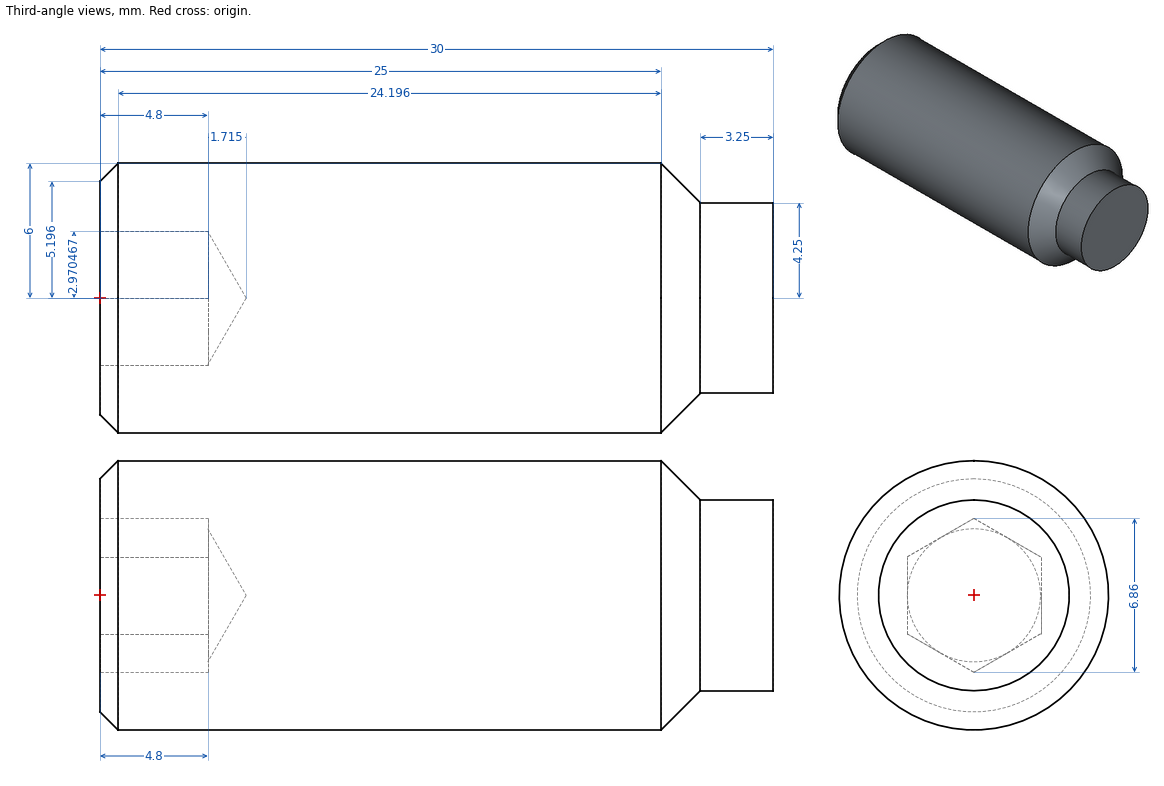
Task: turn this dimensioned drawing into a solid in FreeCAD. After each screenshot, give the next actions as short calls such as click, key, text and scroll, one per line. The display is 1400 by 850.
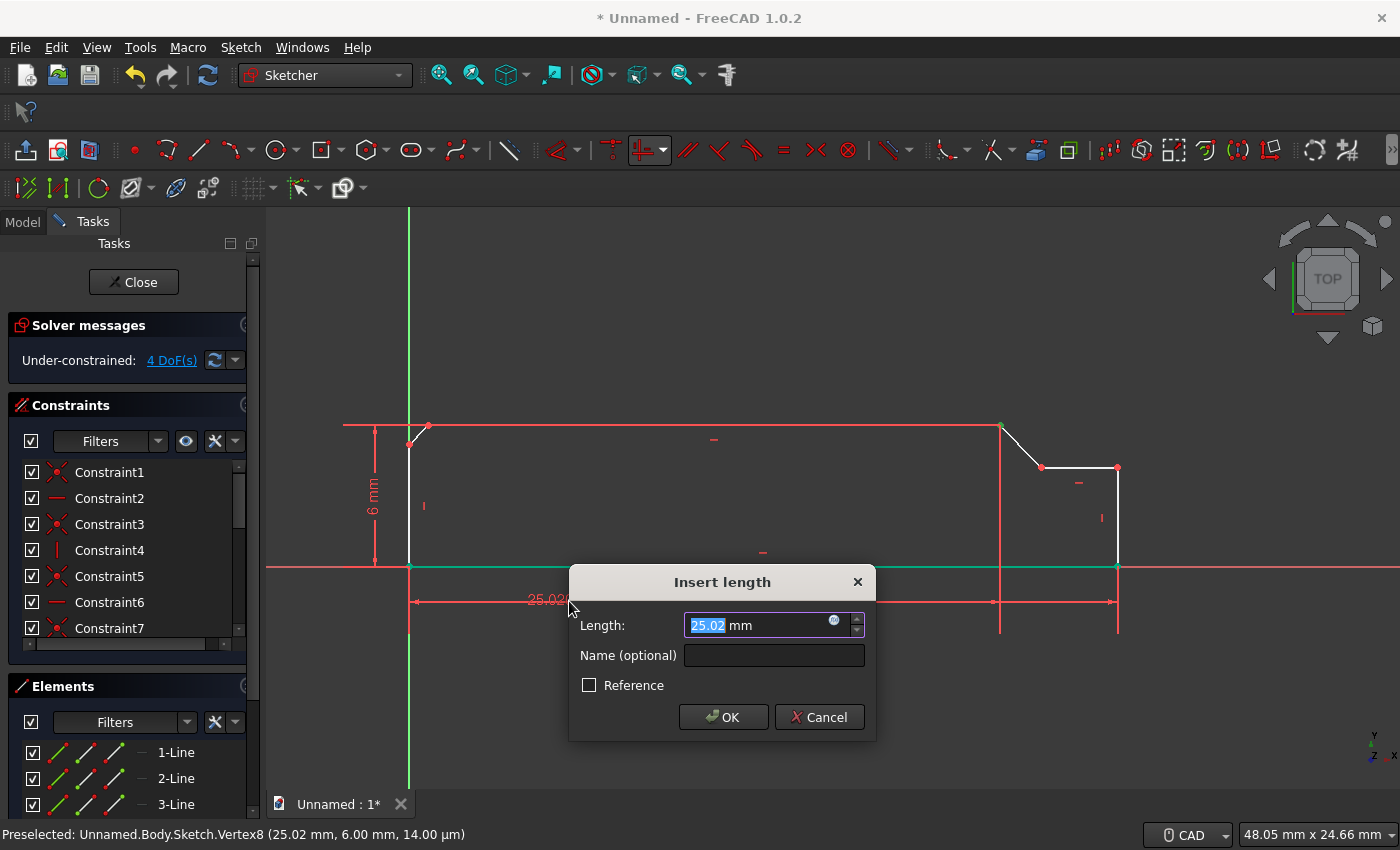
text(25)
key(Return)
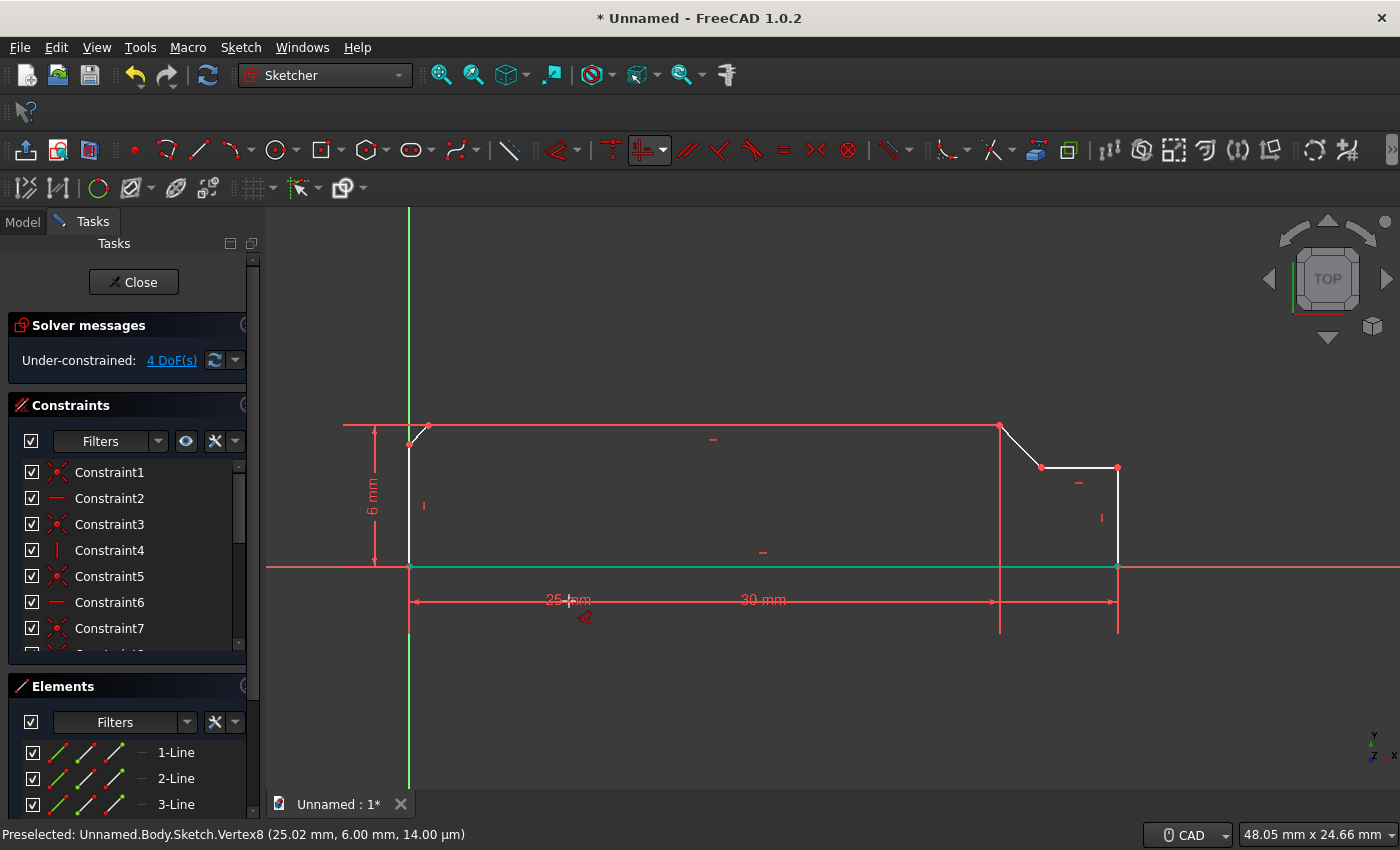
click(1118, 537)
click(1152, 517)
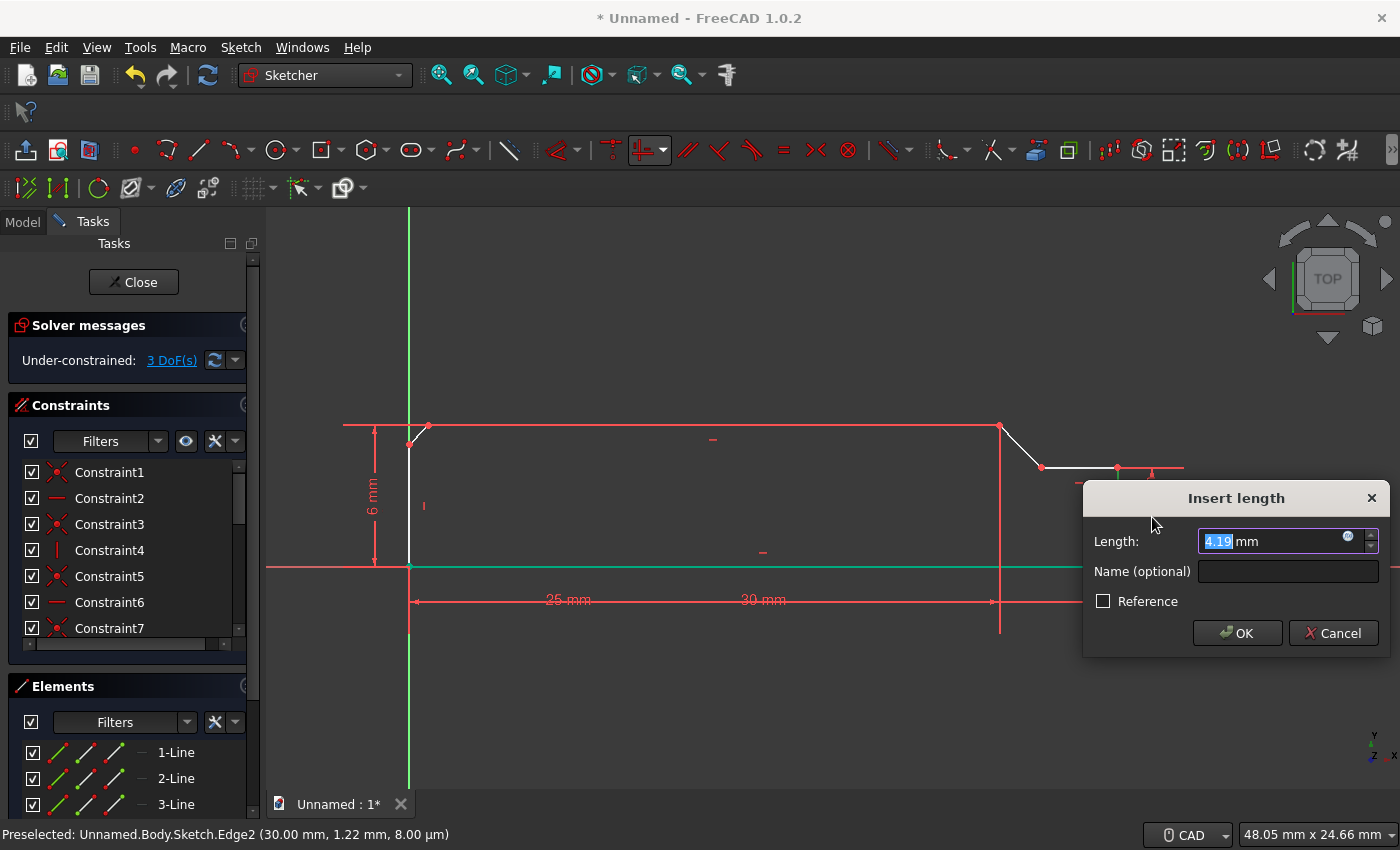
text(4.25)
key(Return)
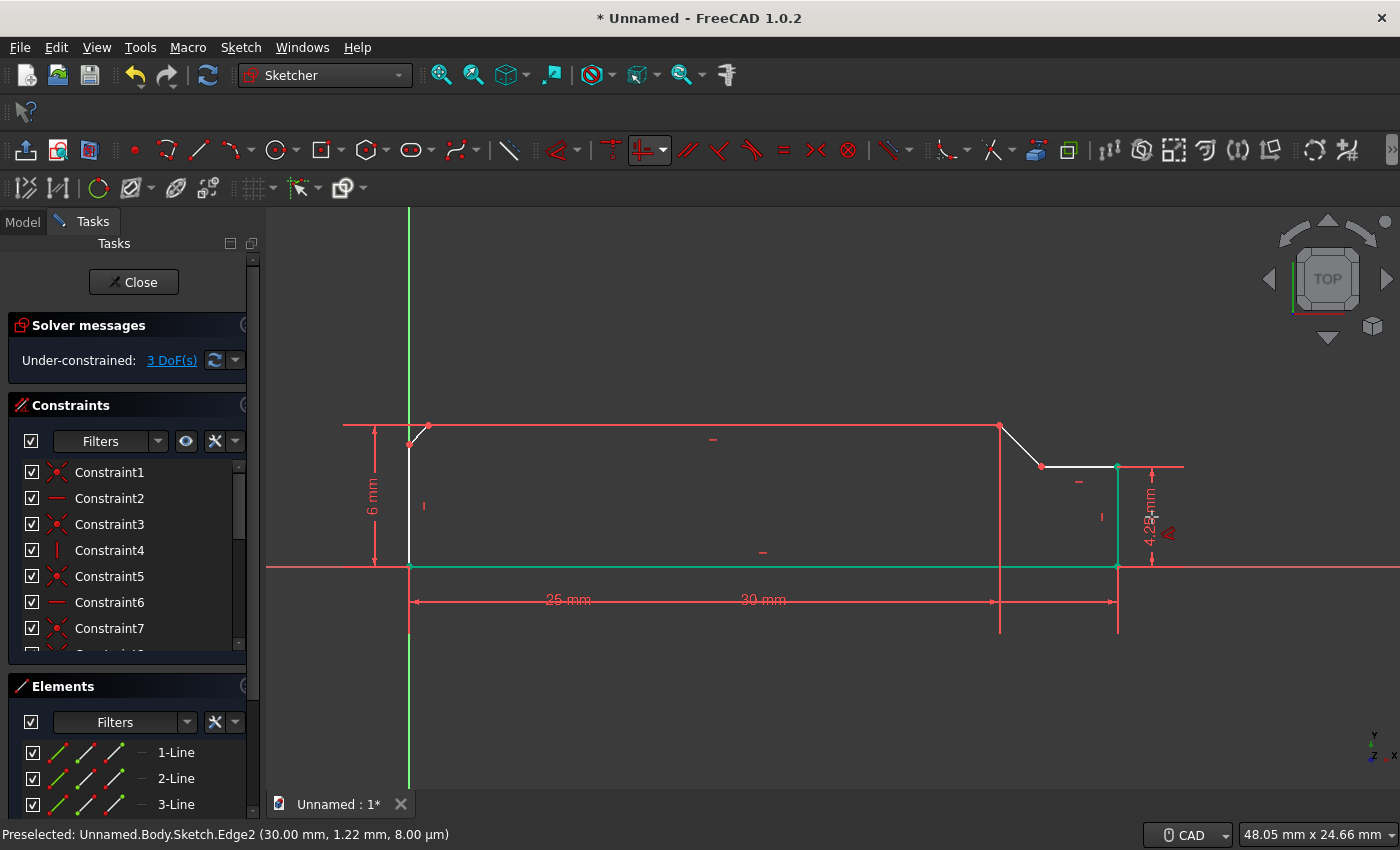
click(1095, 467)
click(1079, 433)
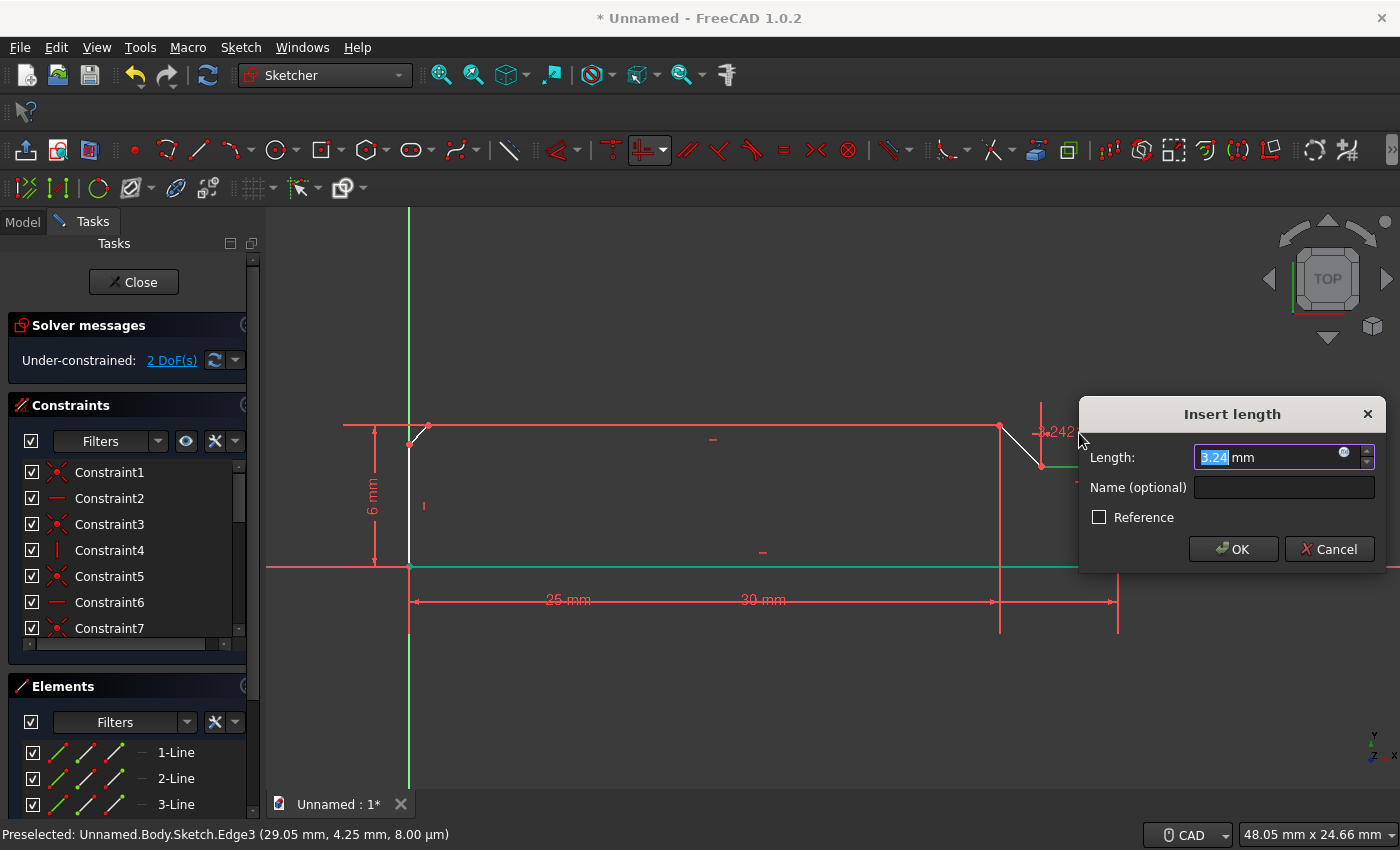
text(3.25)
key(Return)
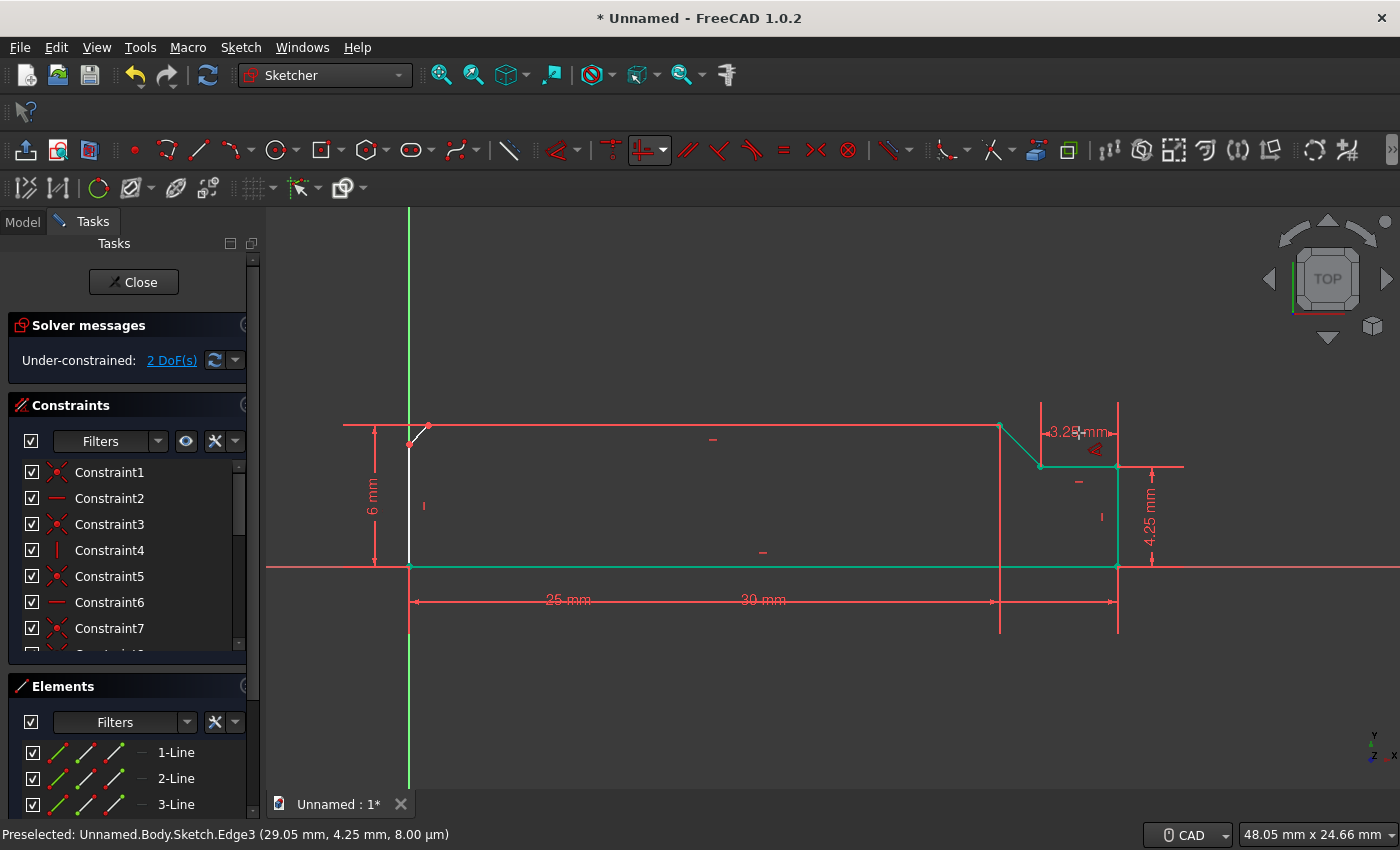
click(409, 482)
click(375, 534)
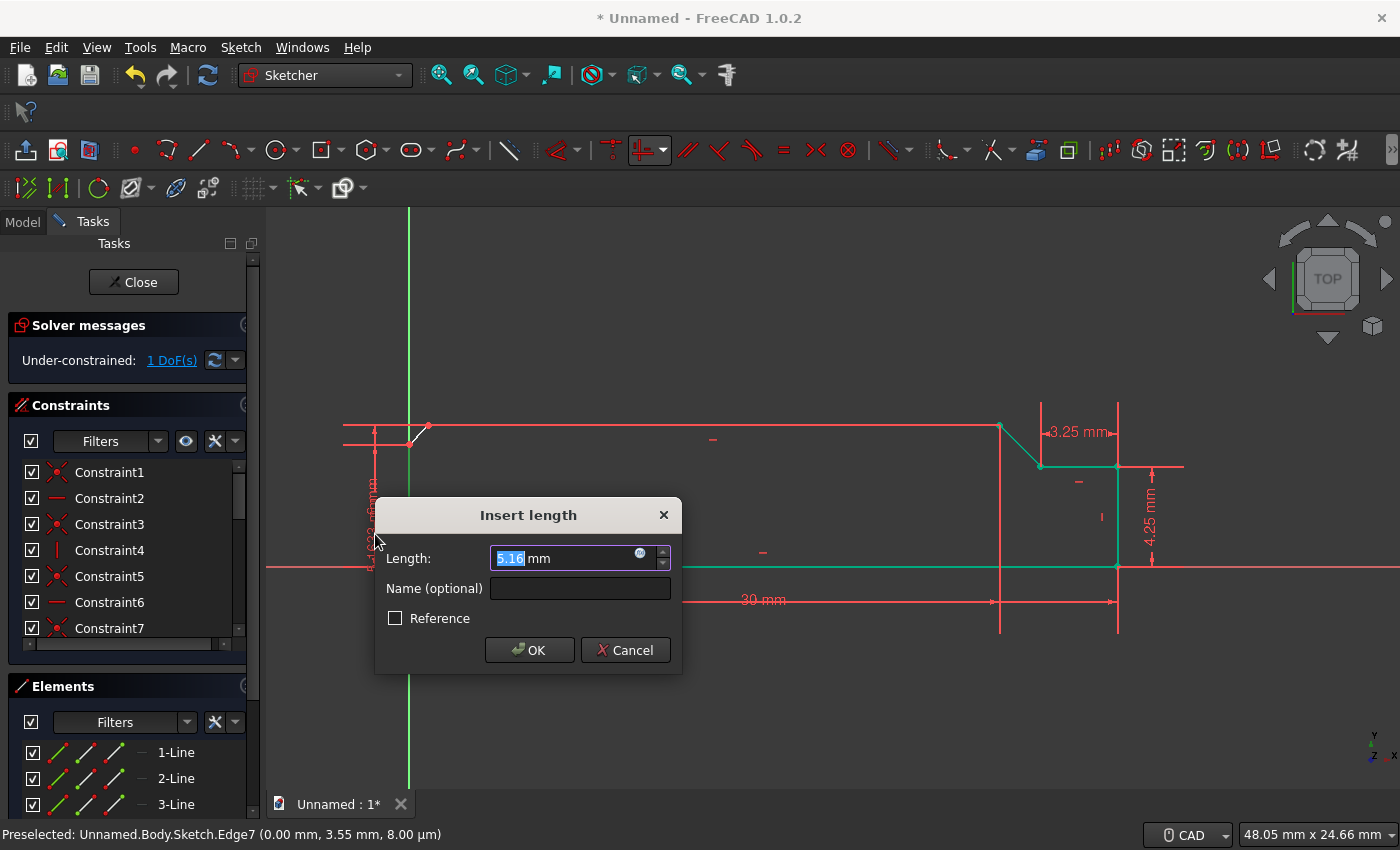
text(5.196)
key(Return)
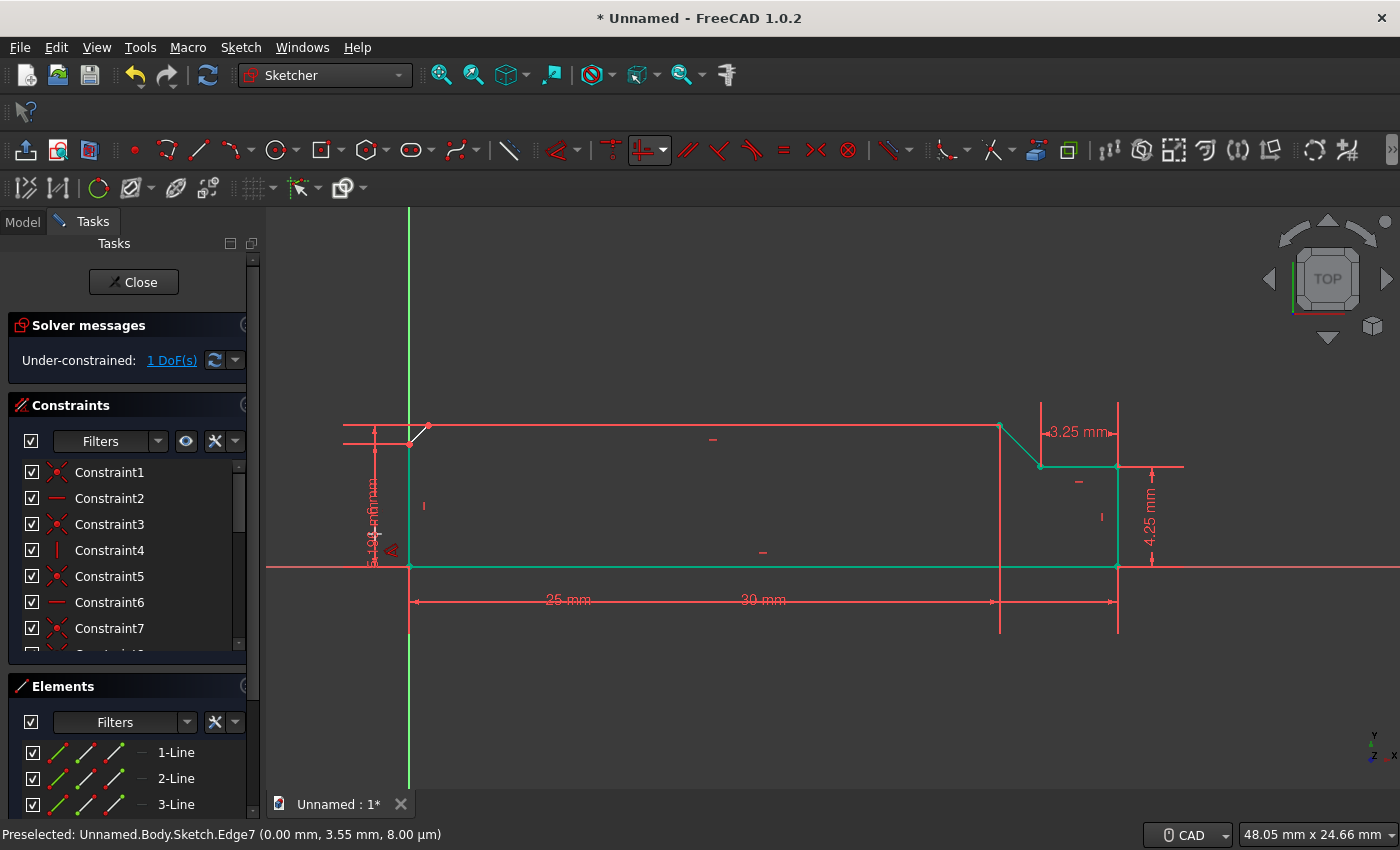
click(828, 425)
click(714, 391)